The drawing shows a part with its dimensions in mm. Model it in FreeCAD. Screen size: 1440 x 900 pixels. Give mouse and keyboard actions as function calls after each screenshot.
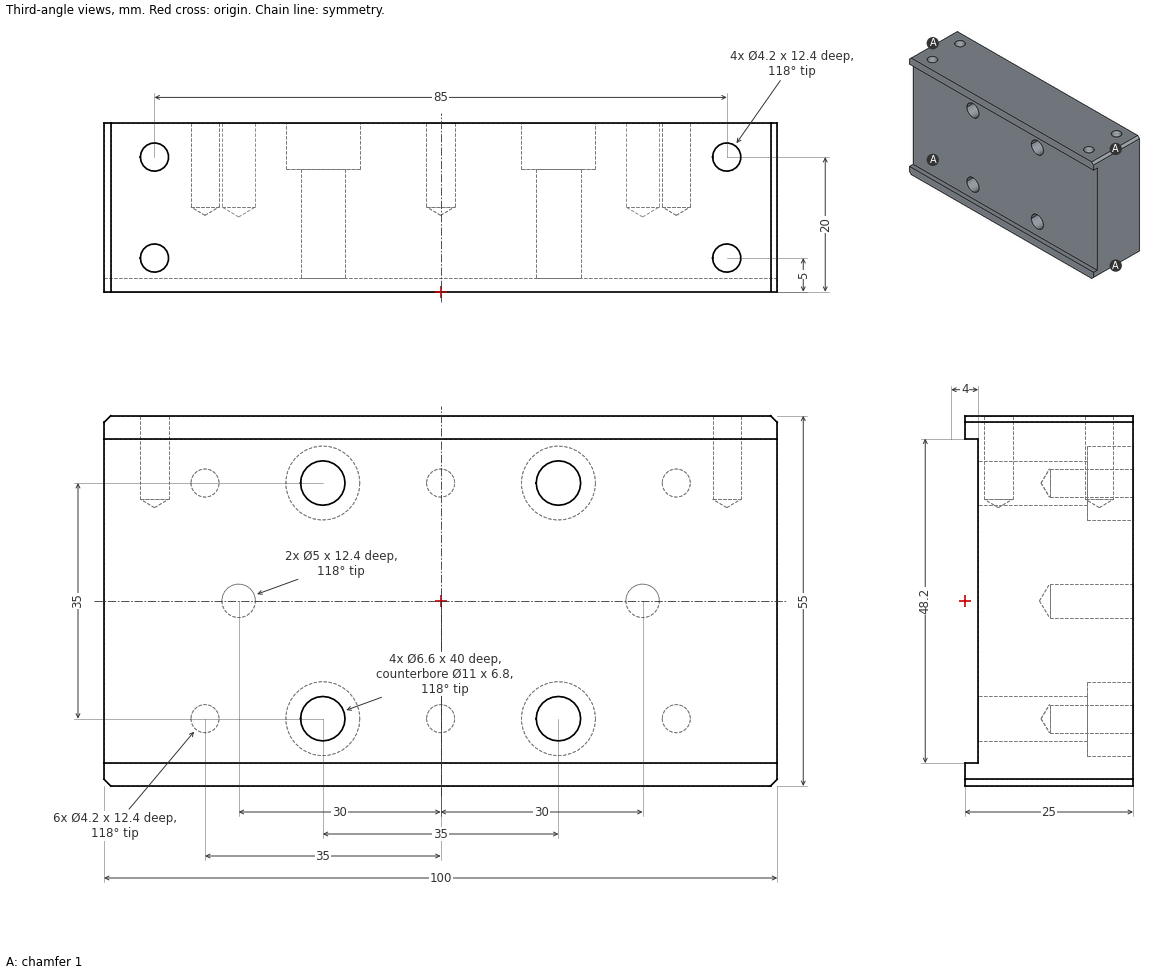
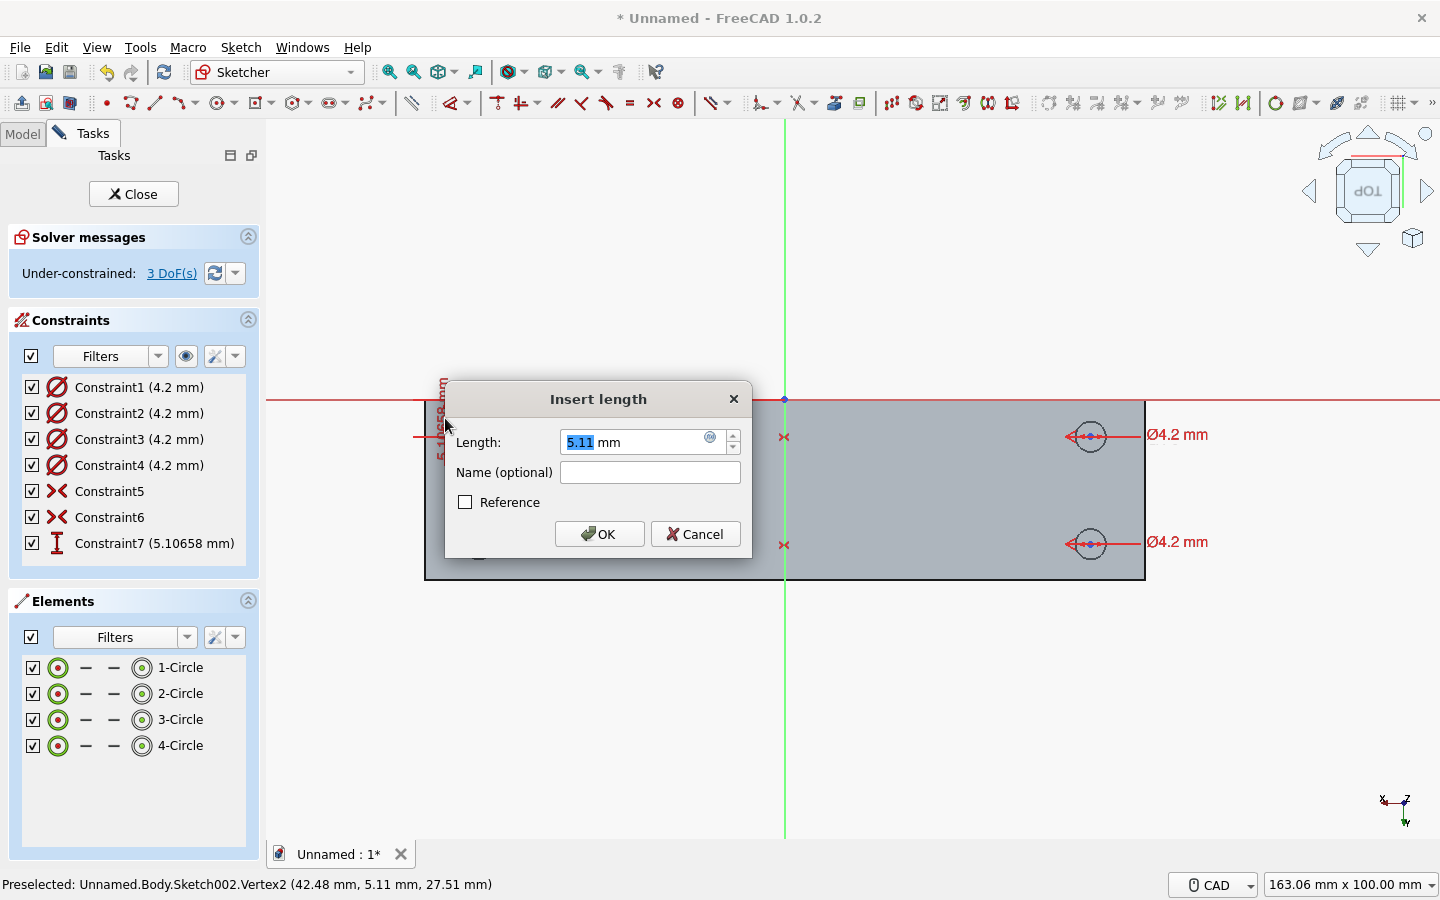
text(5)
key(Return)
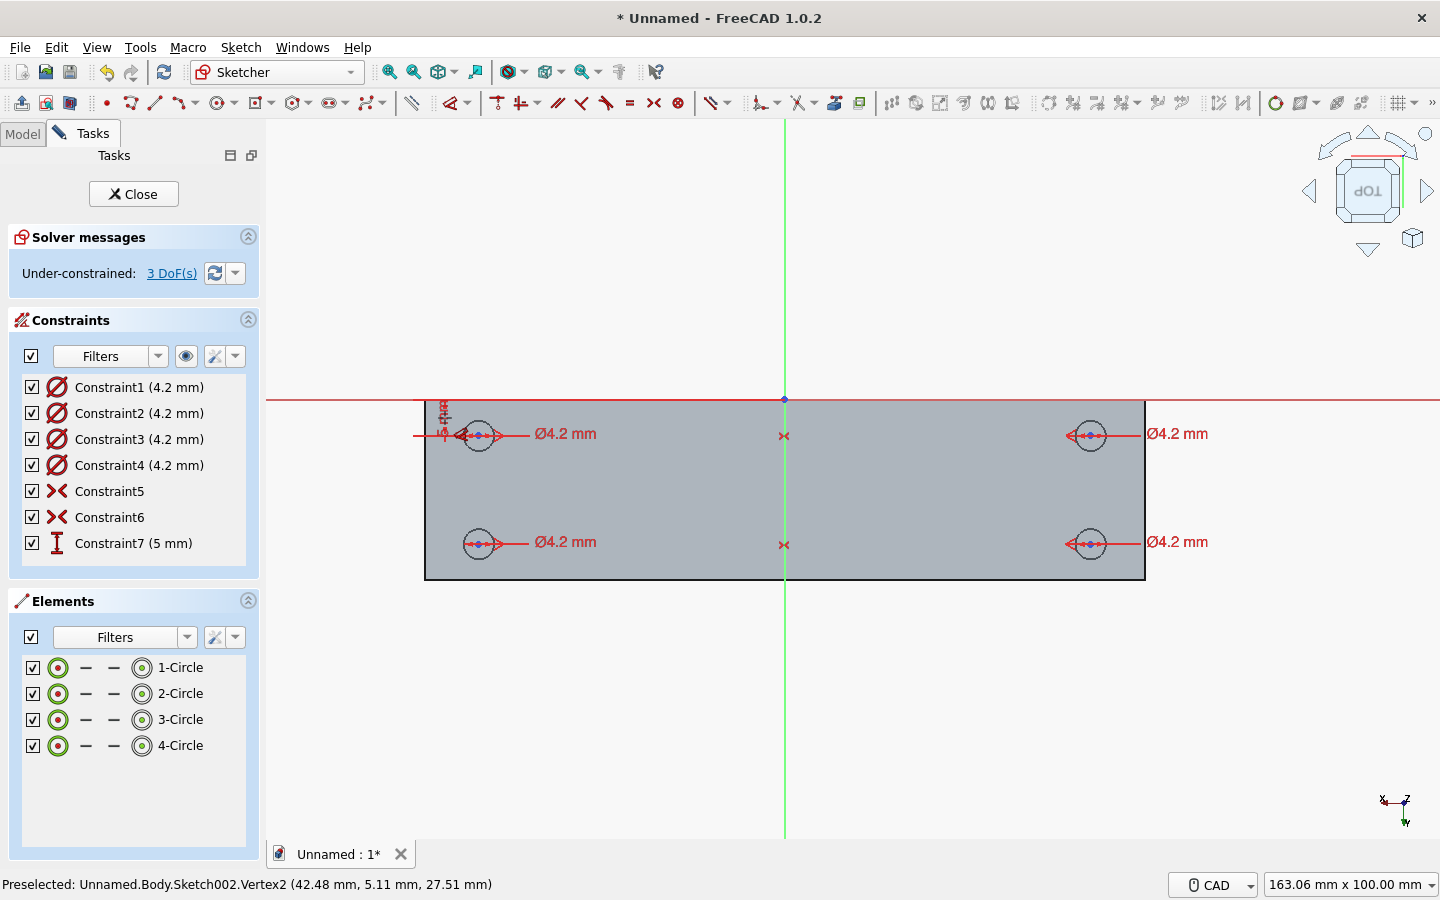
click(479, 544)
click(445, 472)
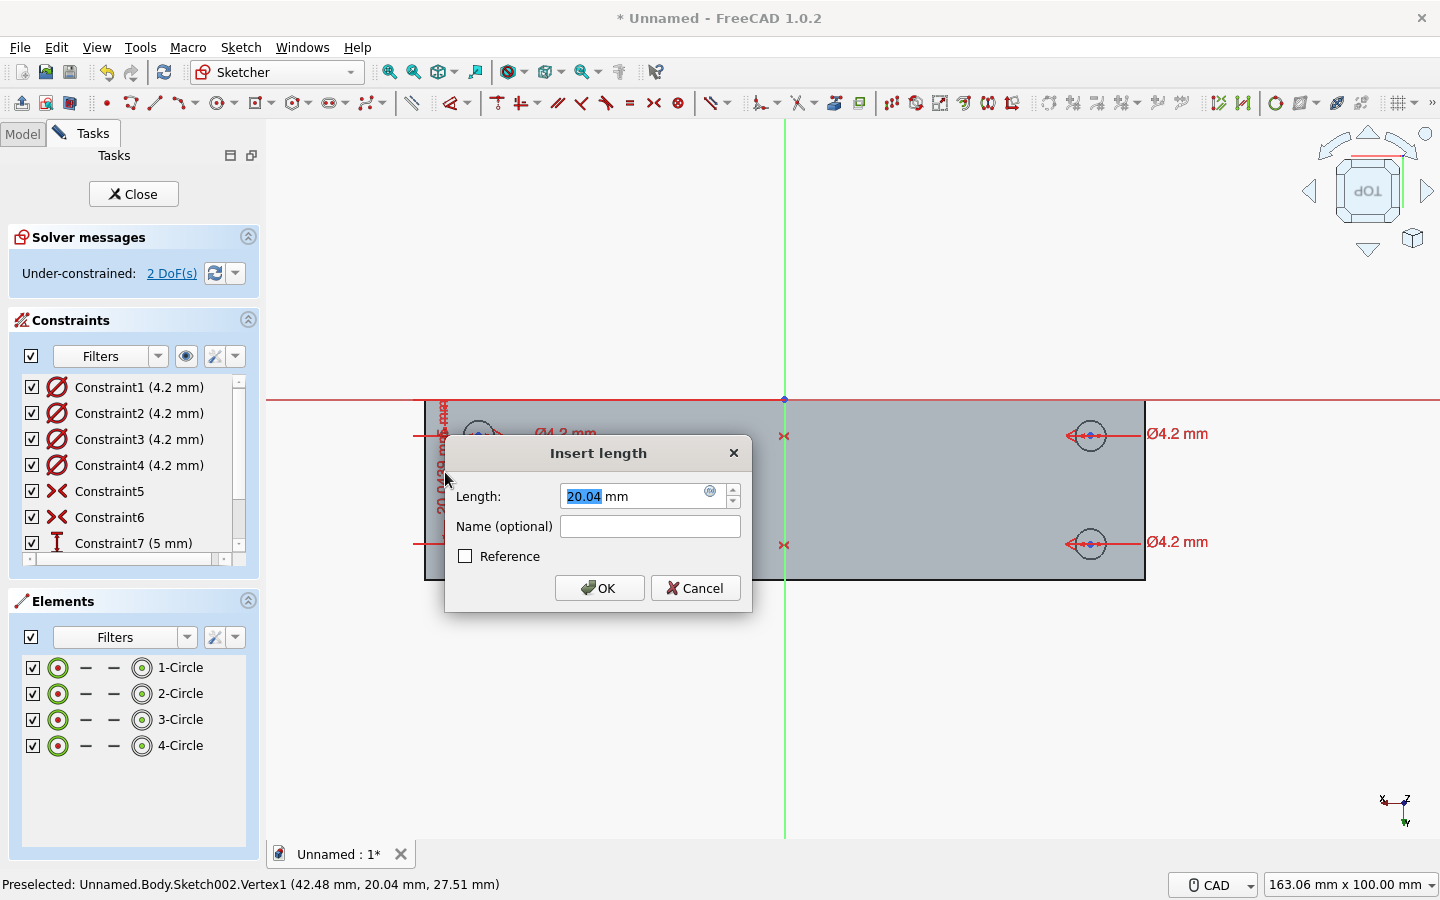
text(20)
key(Return)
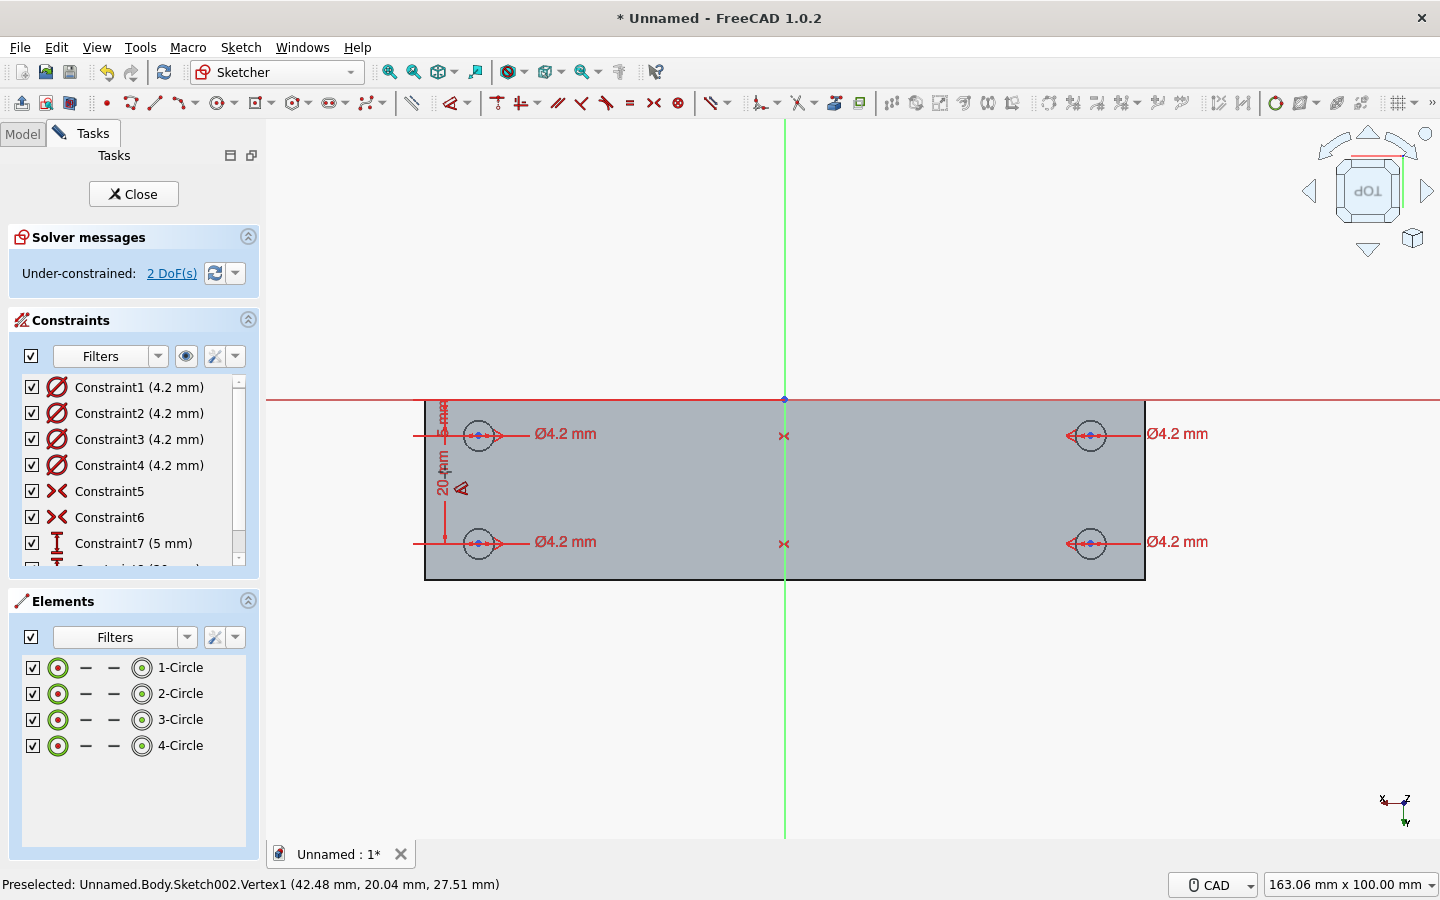
click(479, 544)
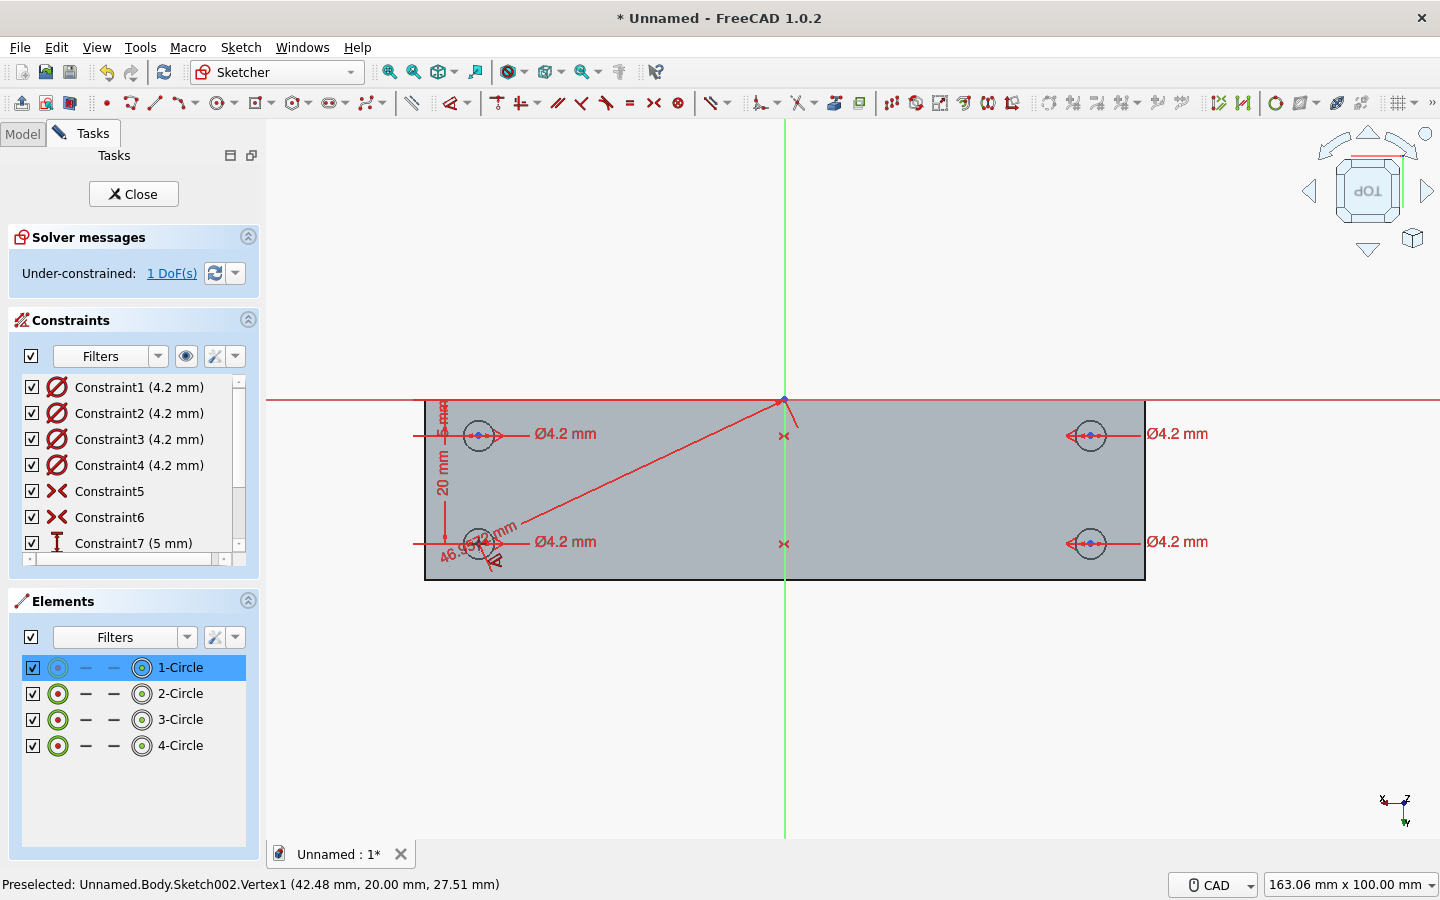
click(1091, 544)
click(644, 578)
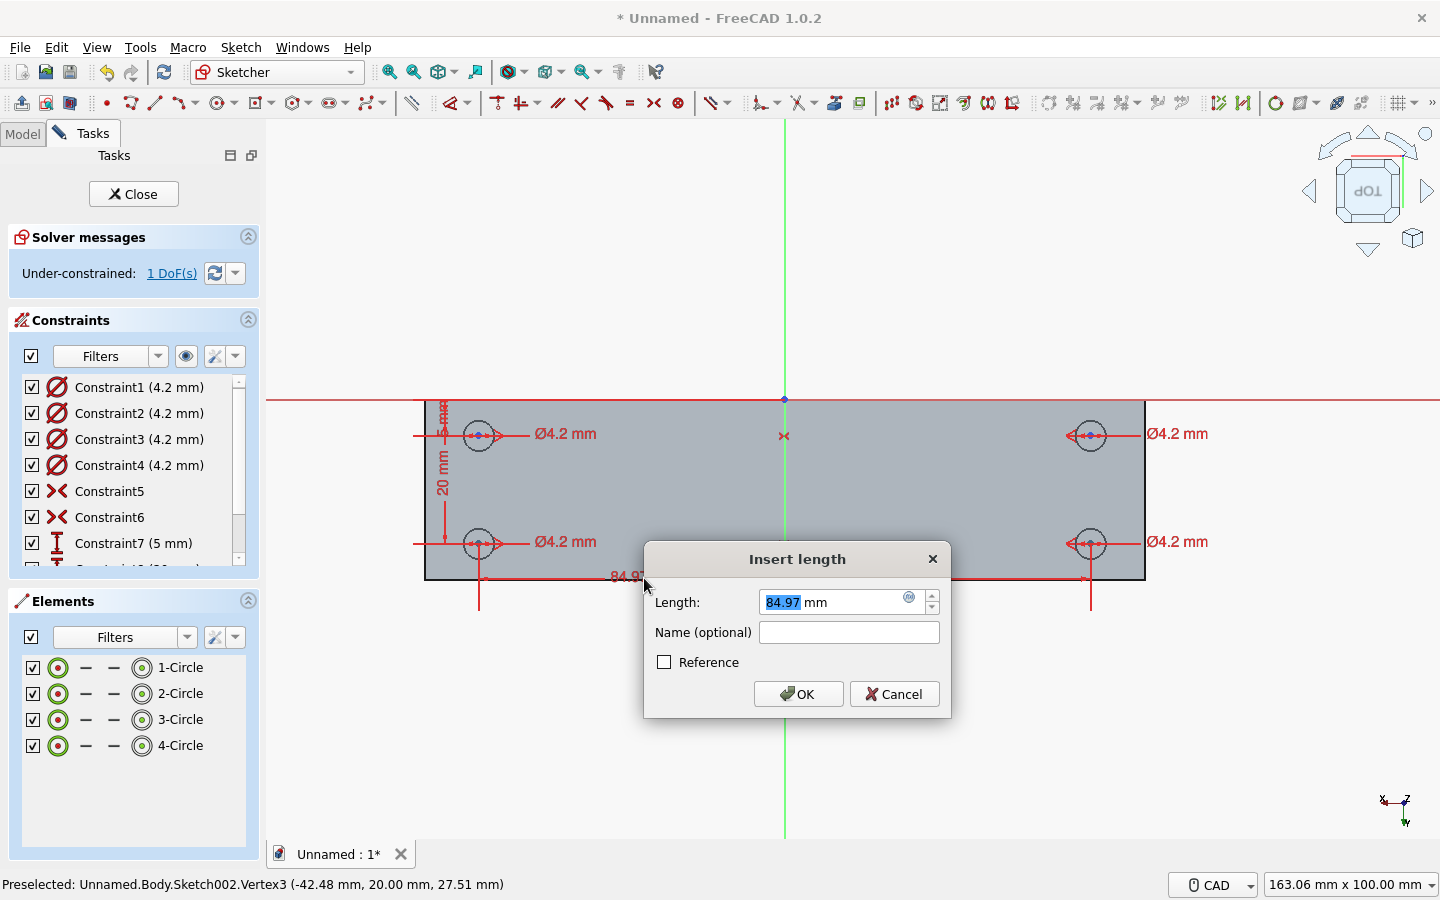
text(85)
key(Return)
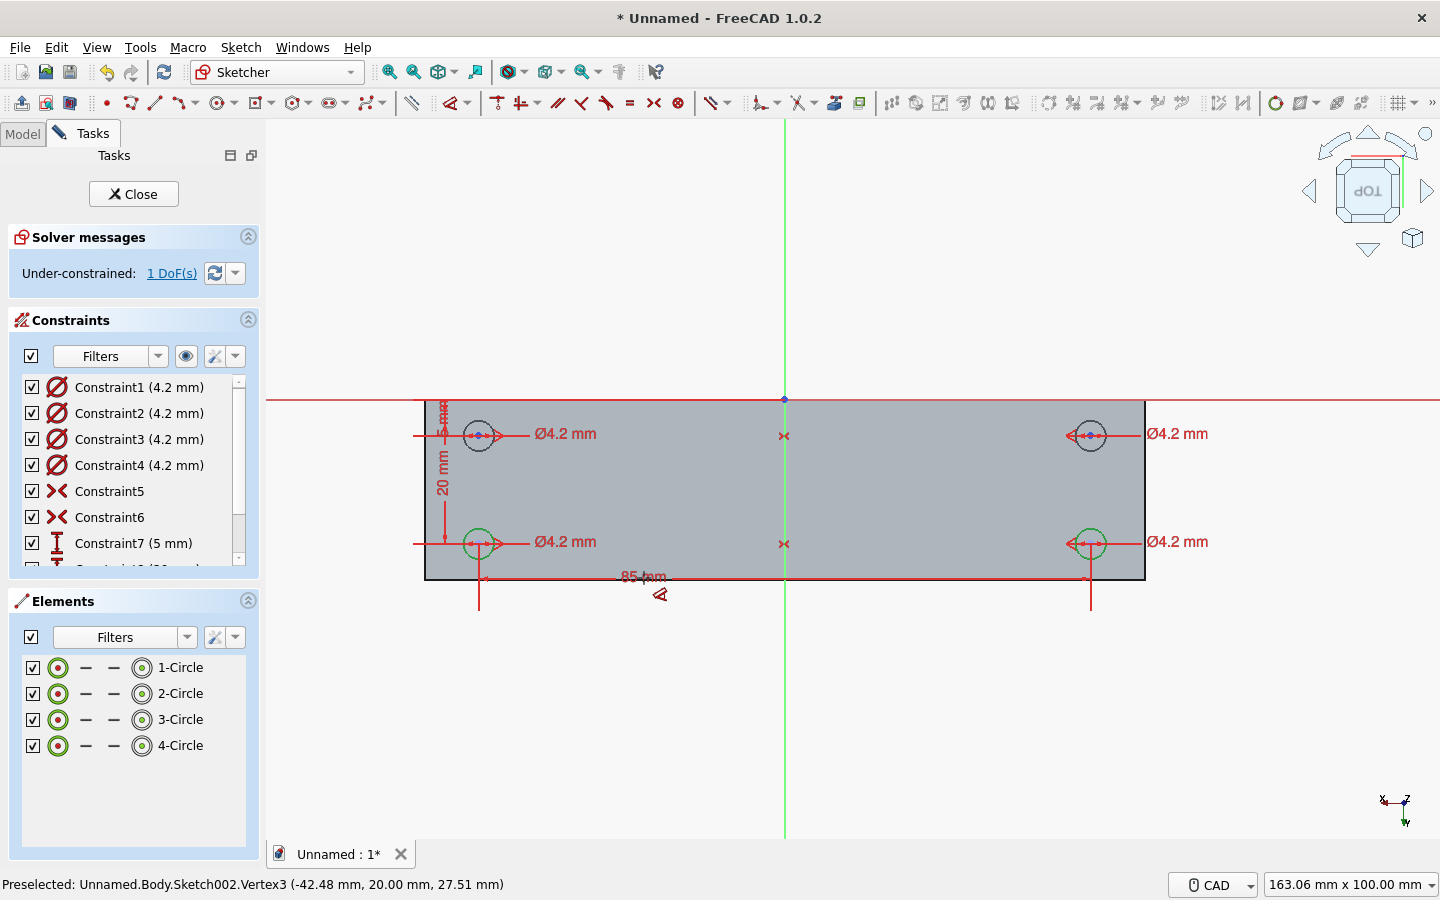
click(479, 436)